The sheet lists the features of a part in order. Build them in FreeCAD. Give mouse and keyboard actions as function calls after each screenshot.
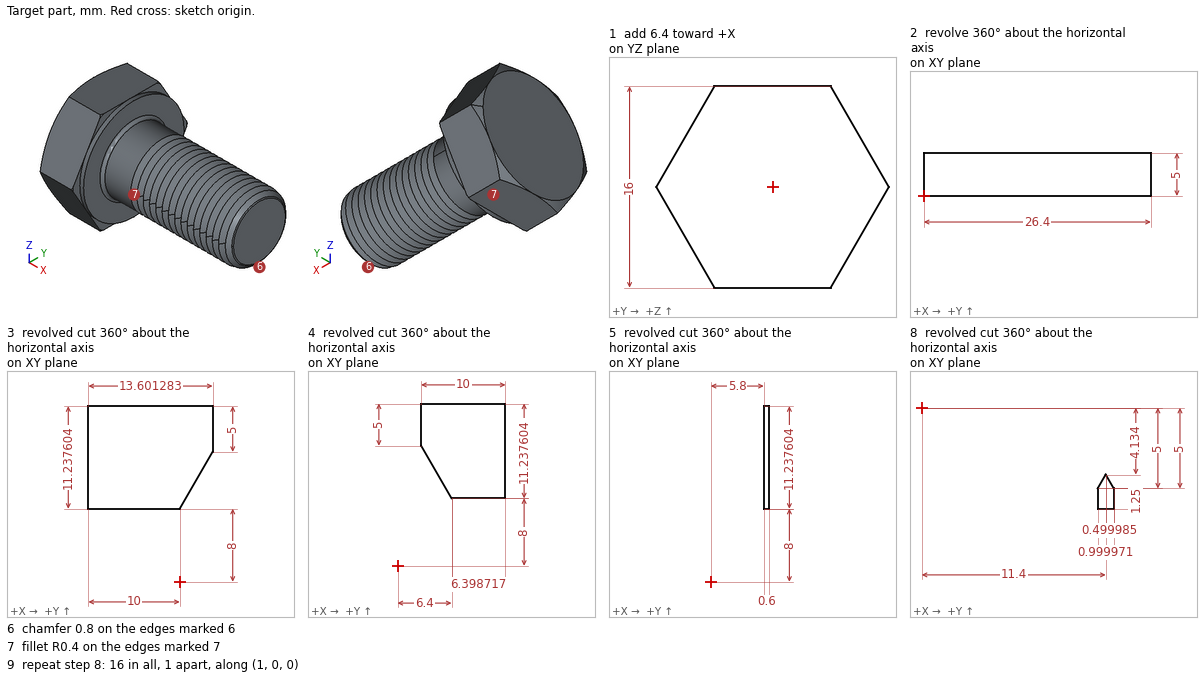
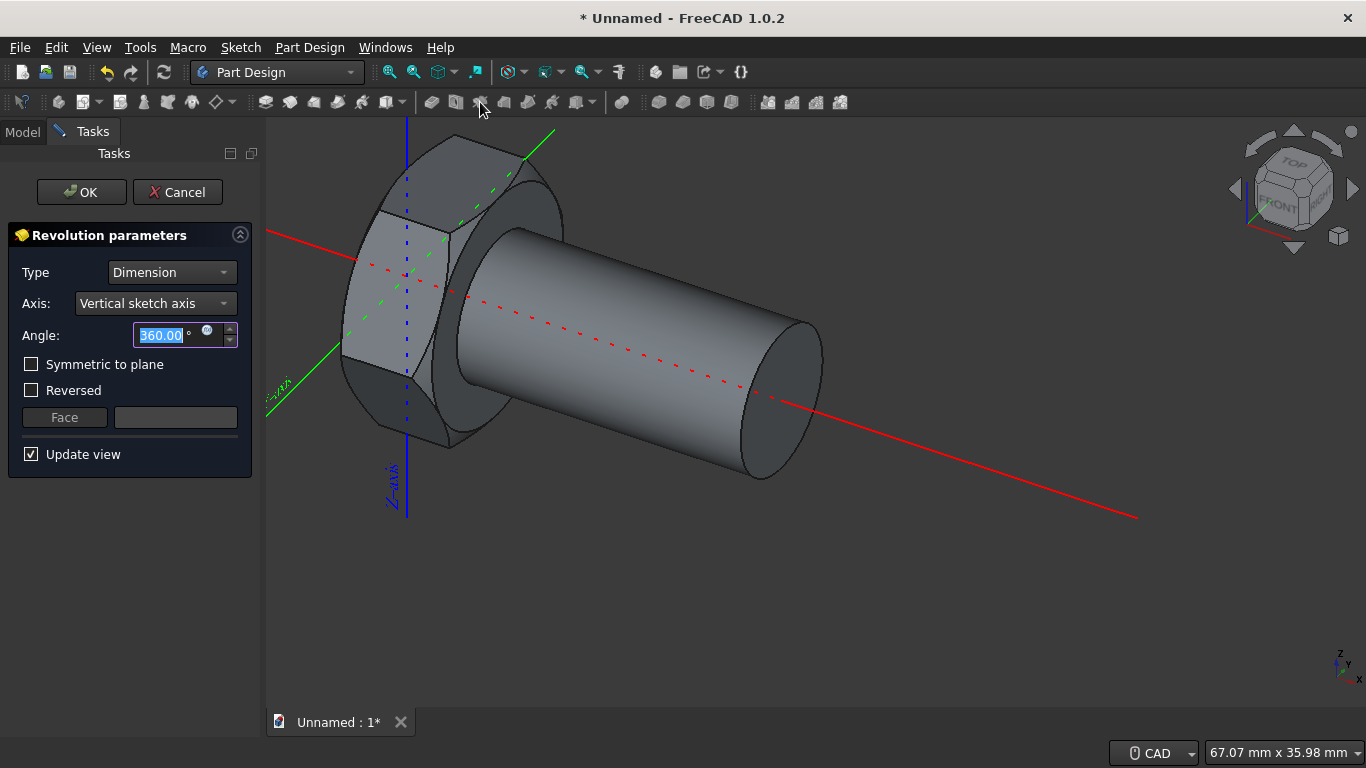
click(156, 304)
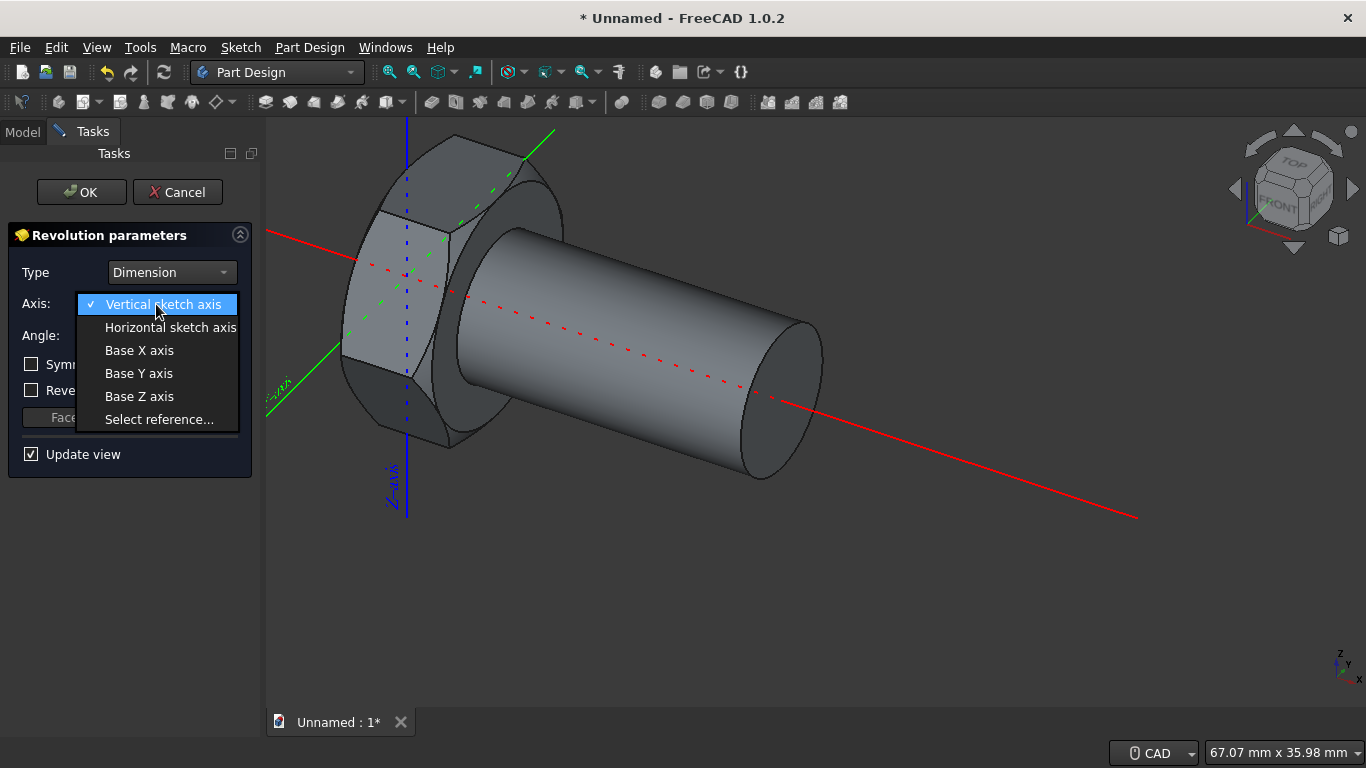
click(156, 328)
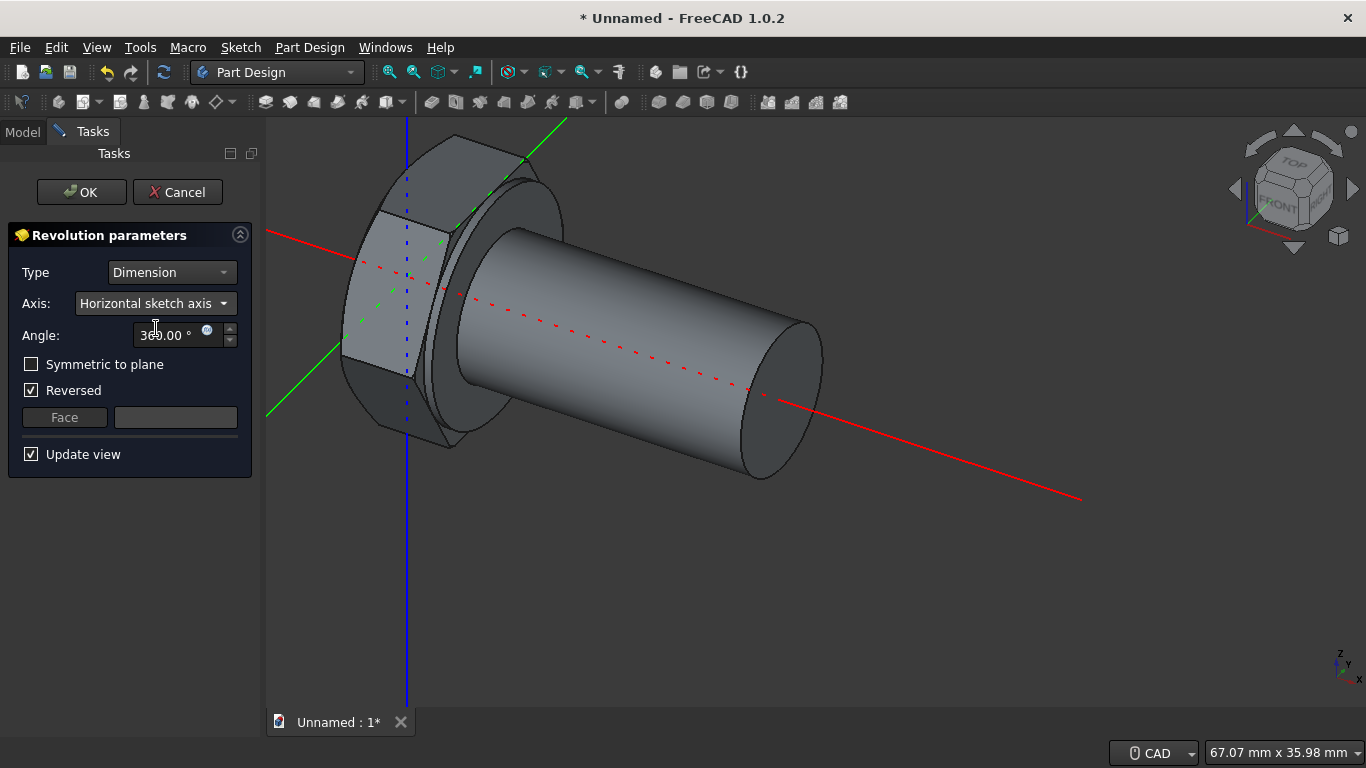
click(82, 192)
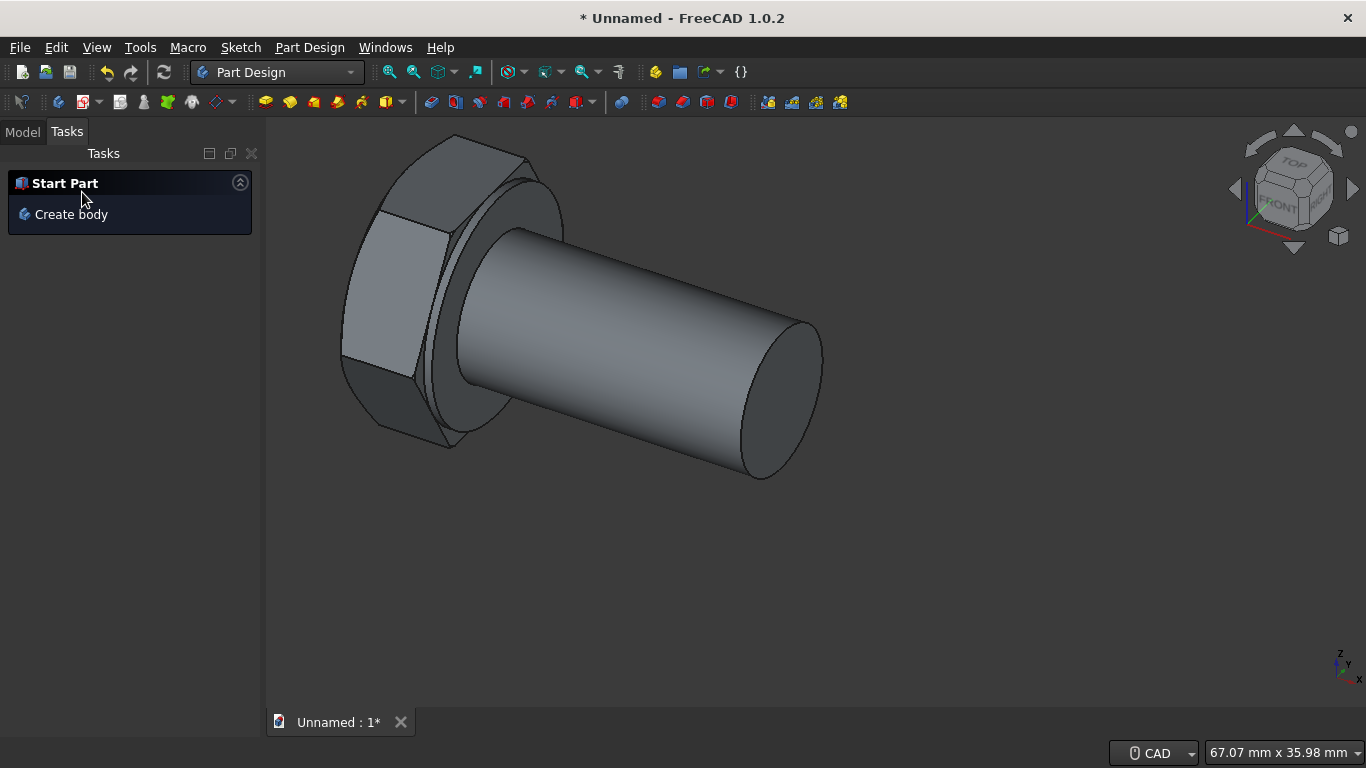
key(v)
key(f)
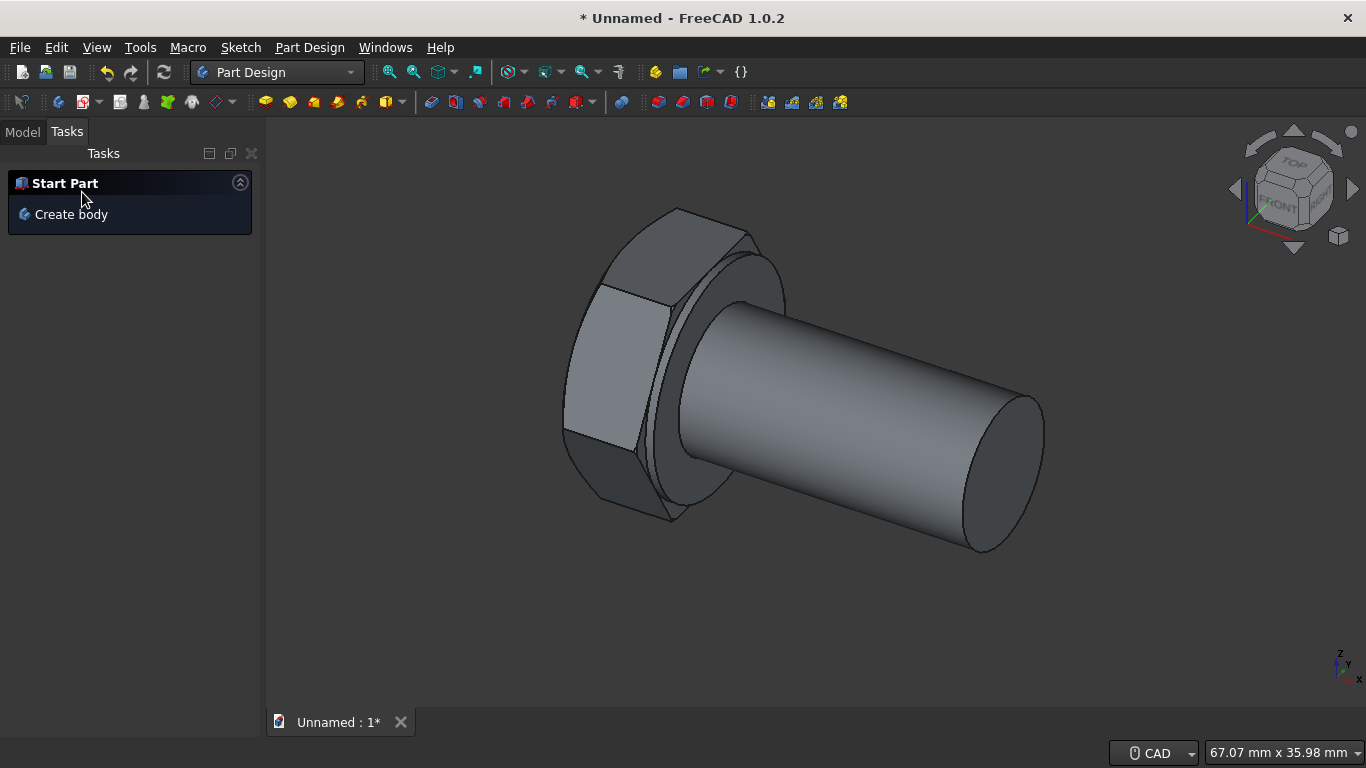
click(962, 514)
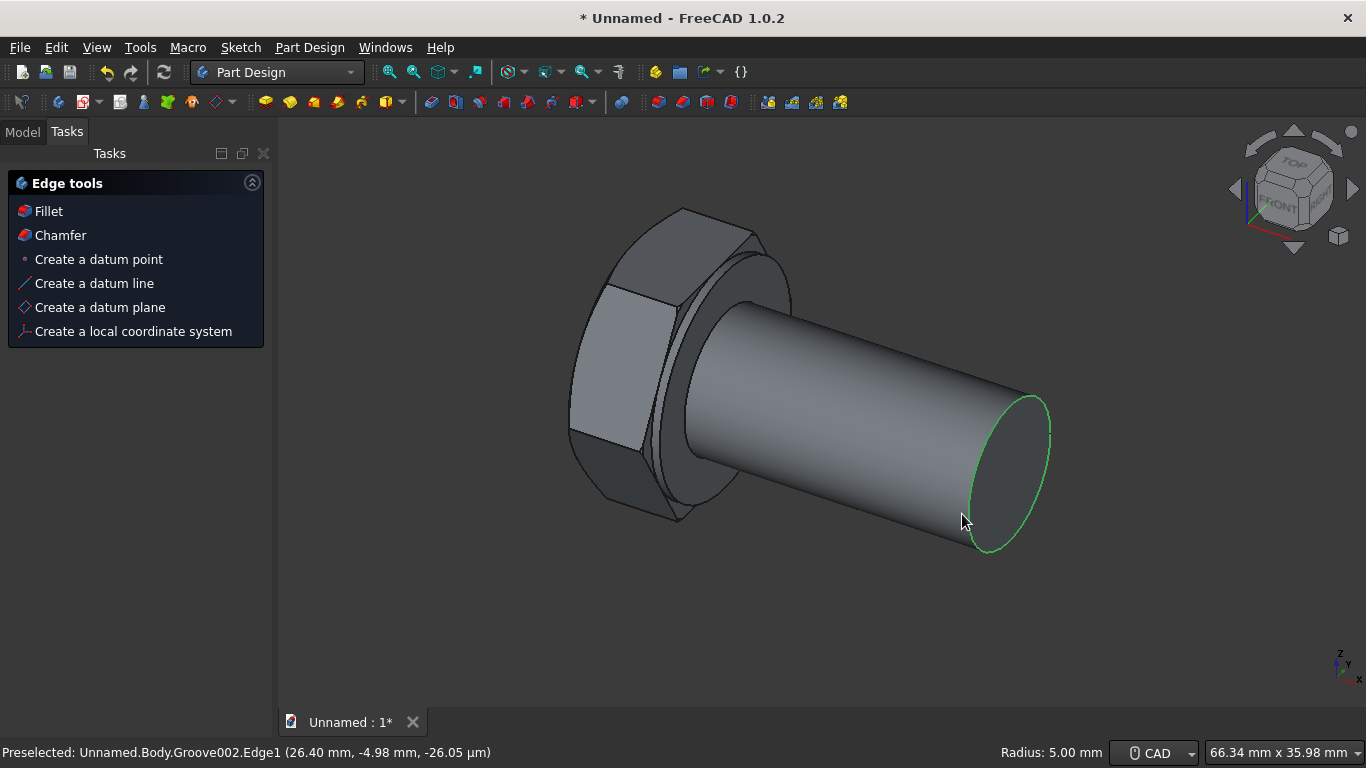
click(684, 102)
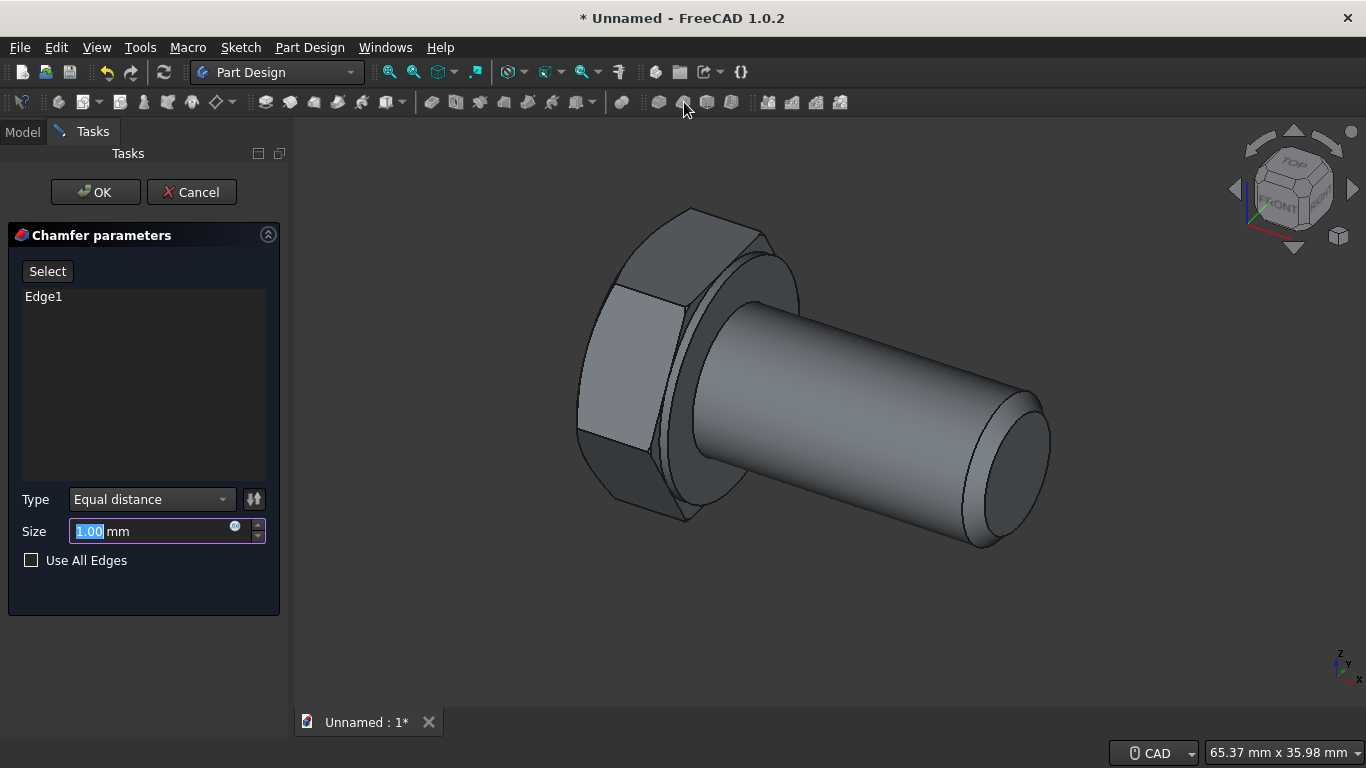
text(0.8)
key(Tab)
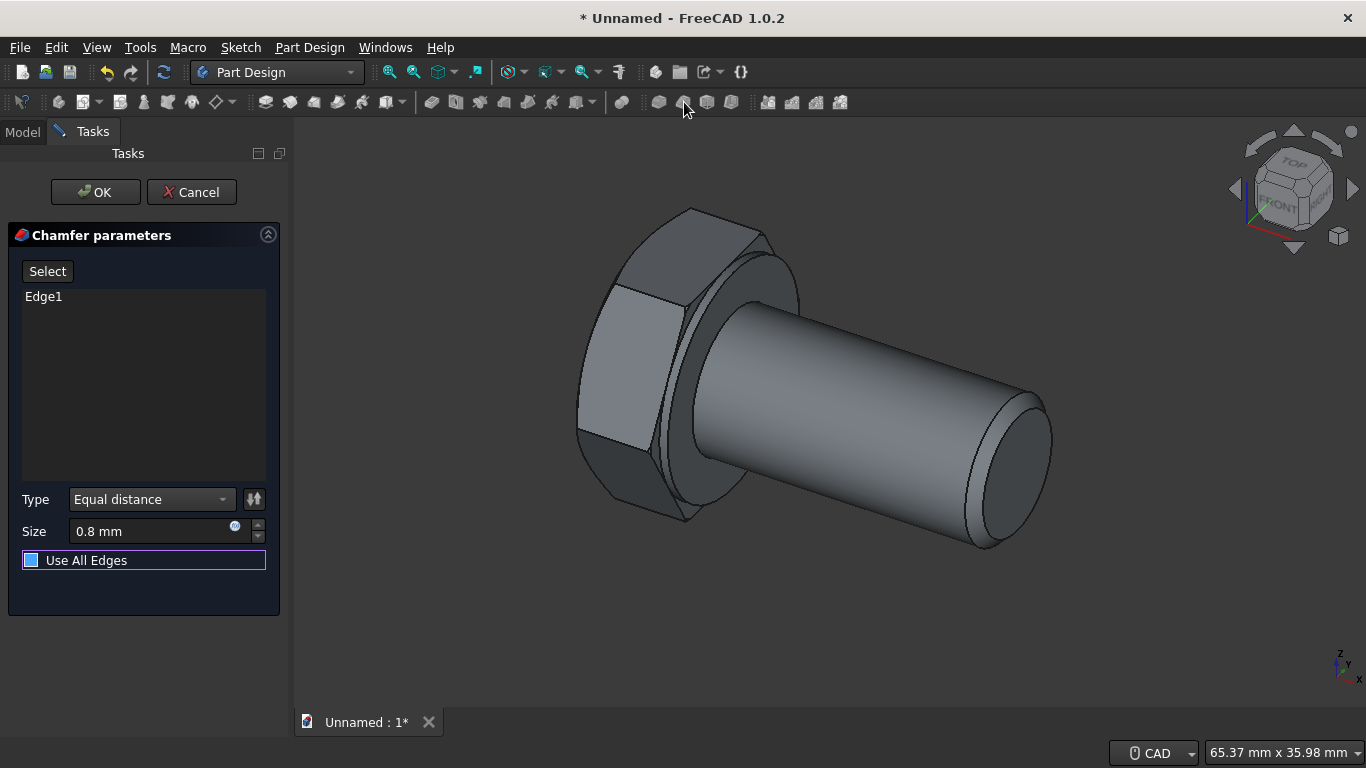
click(96, 192)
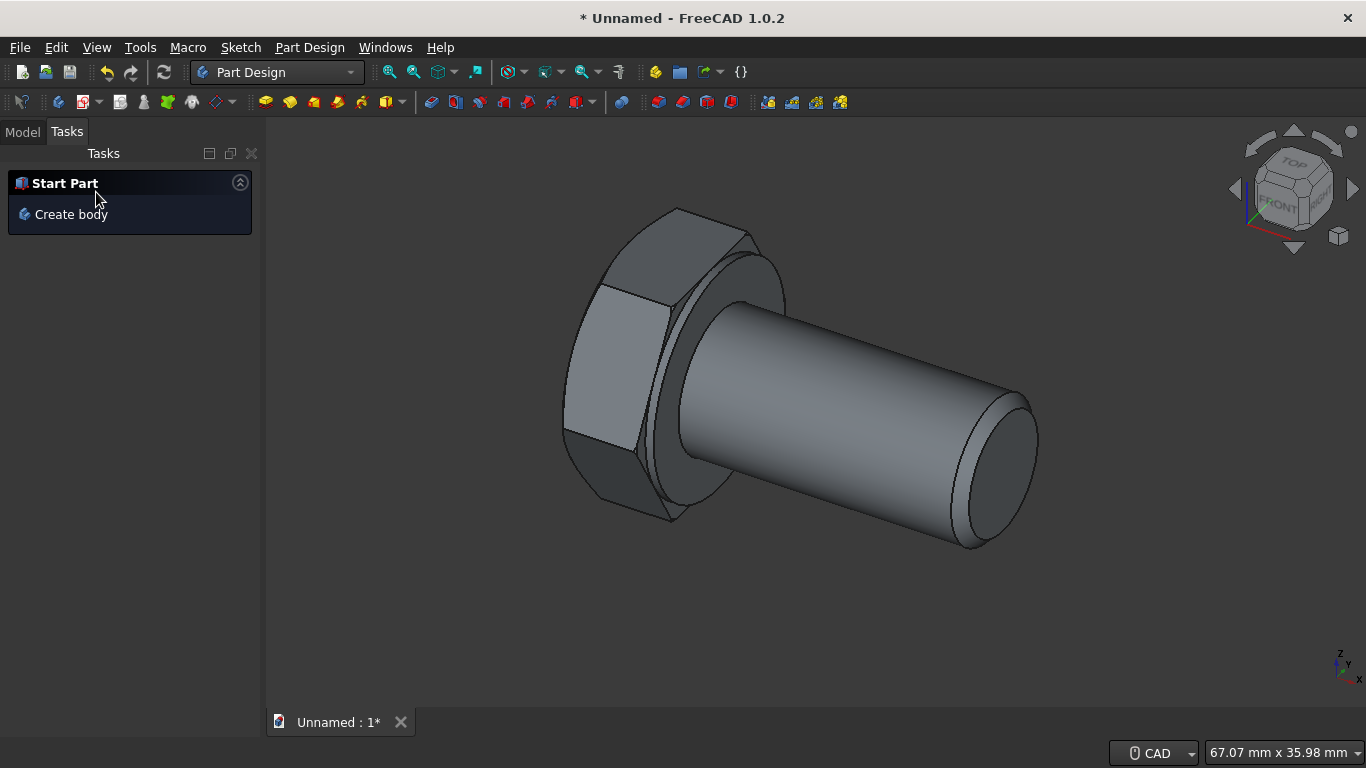
key(0)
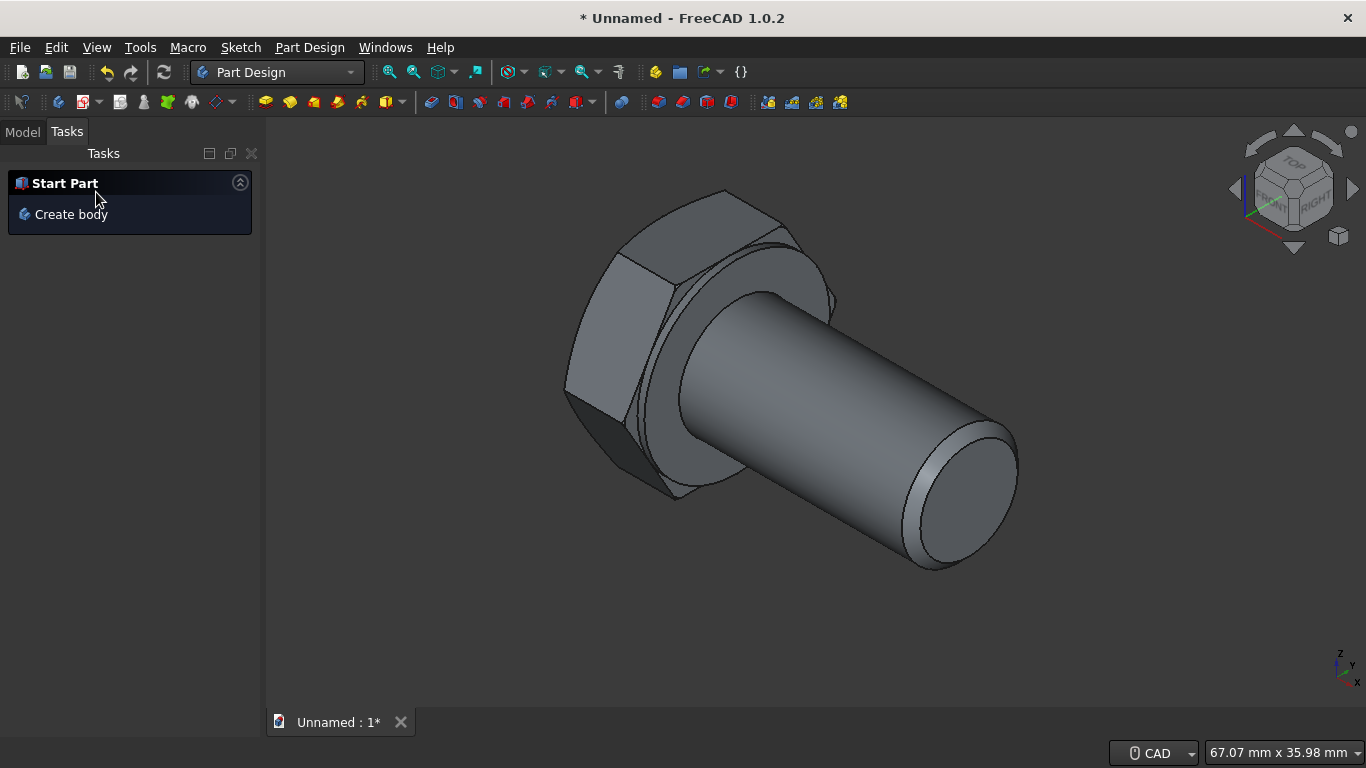
key(2)